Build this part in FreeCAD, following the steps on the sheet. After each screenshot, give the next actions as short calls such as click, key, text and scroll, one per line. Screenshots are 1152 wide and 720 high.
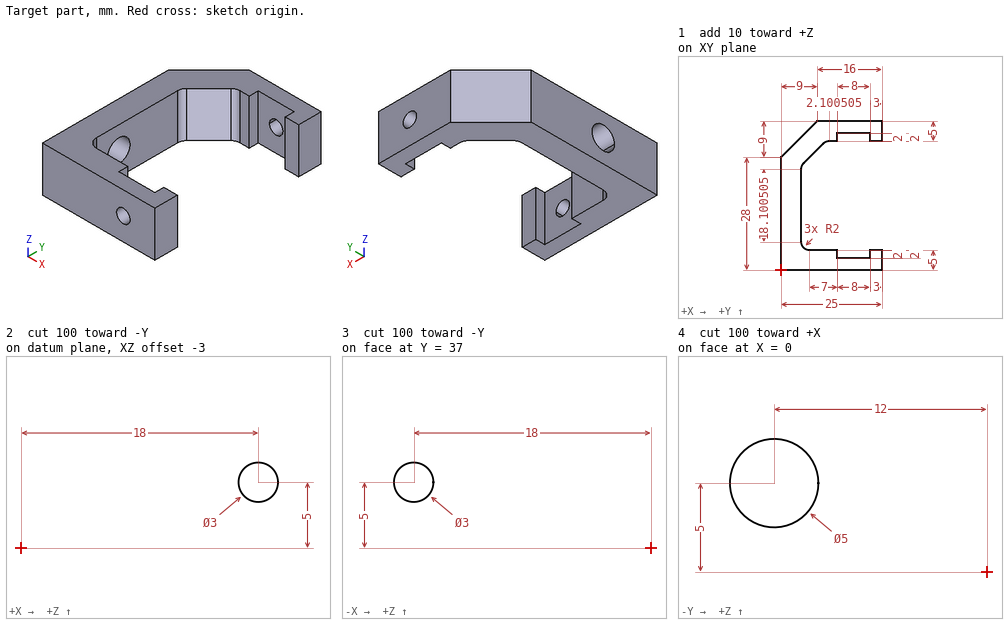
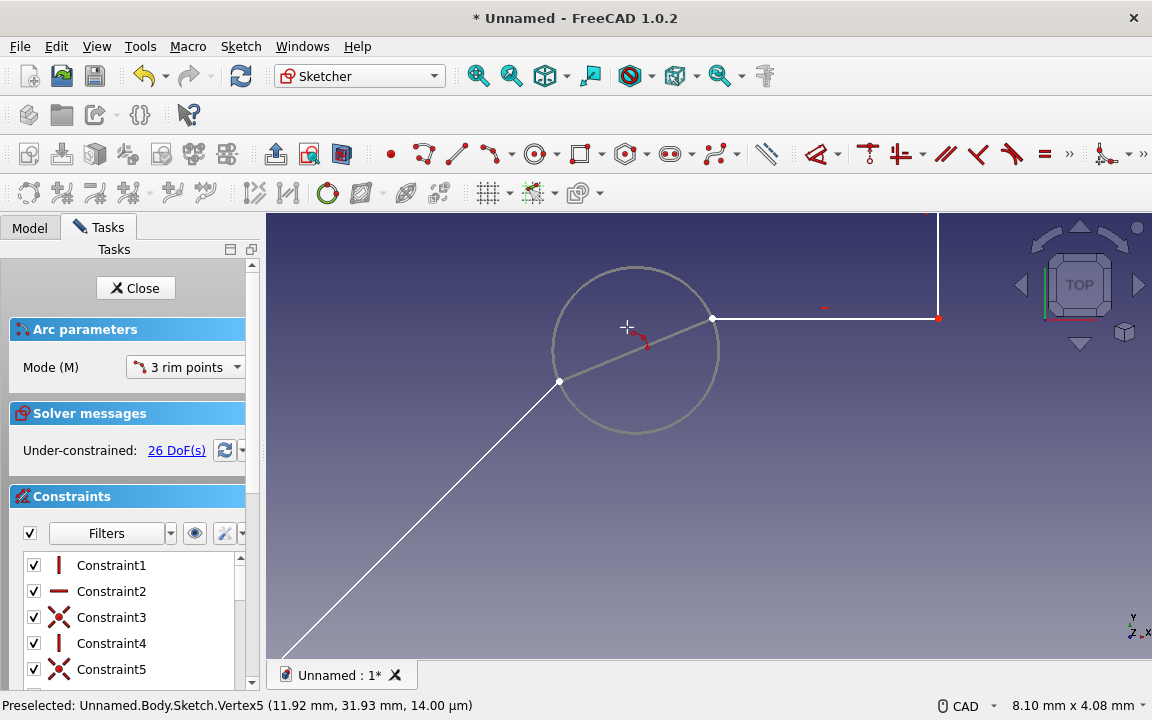
click(627, 328)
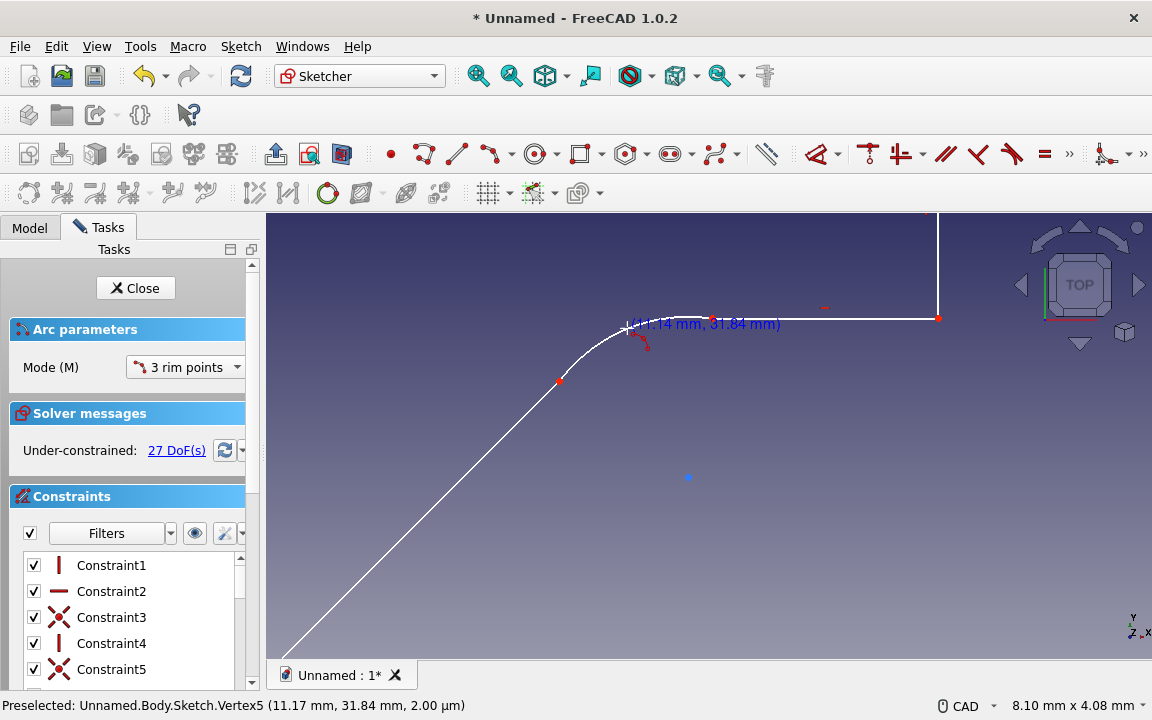
scroll(630, 327, down, 13)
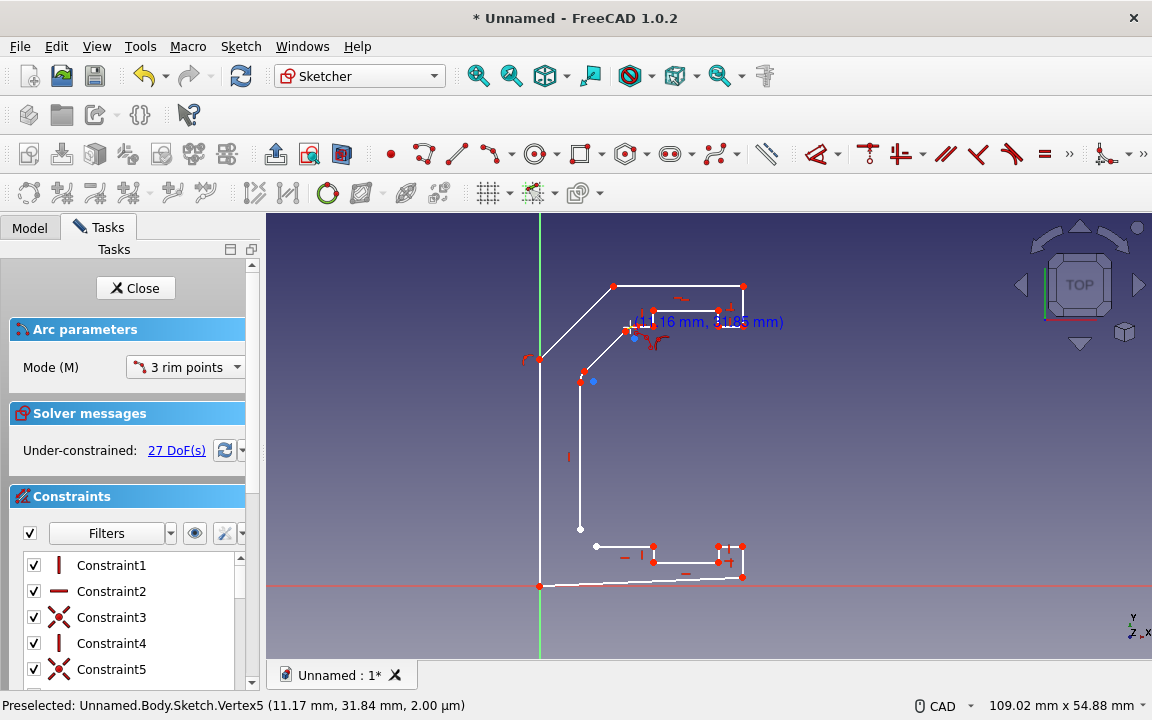
click(597, 547)
click(580, 530)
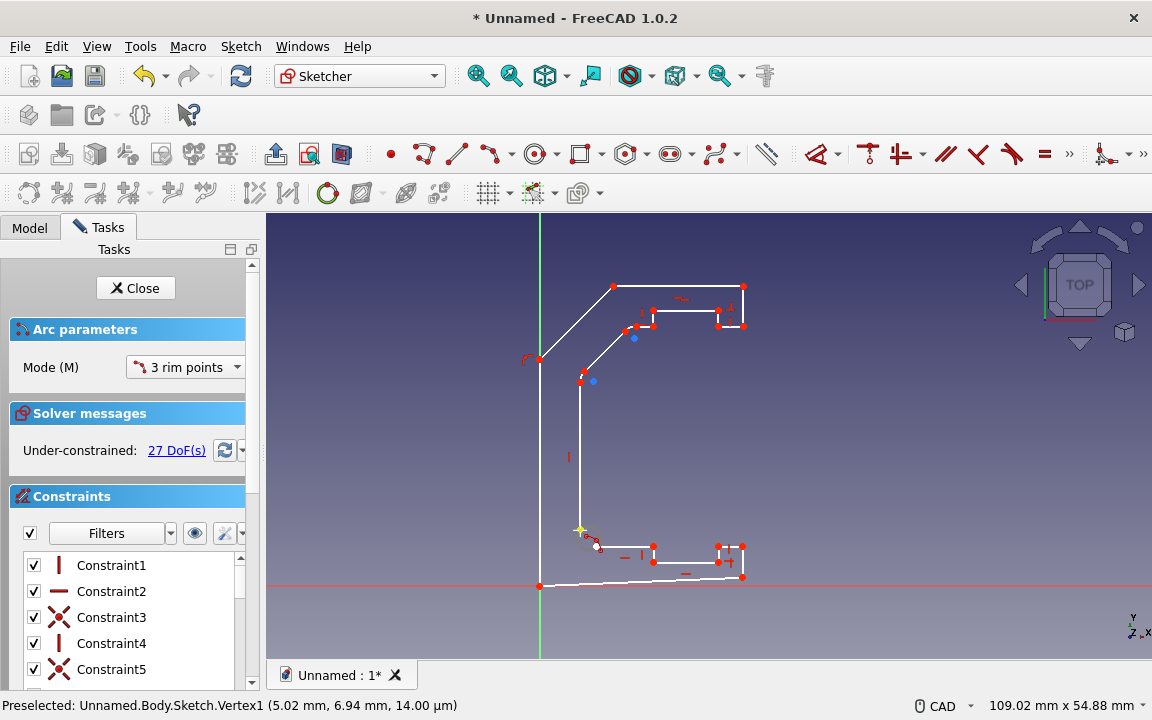
scroll(585, 541, up, 7)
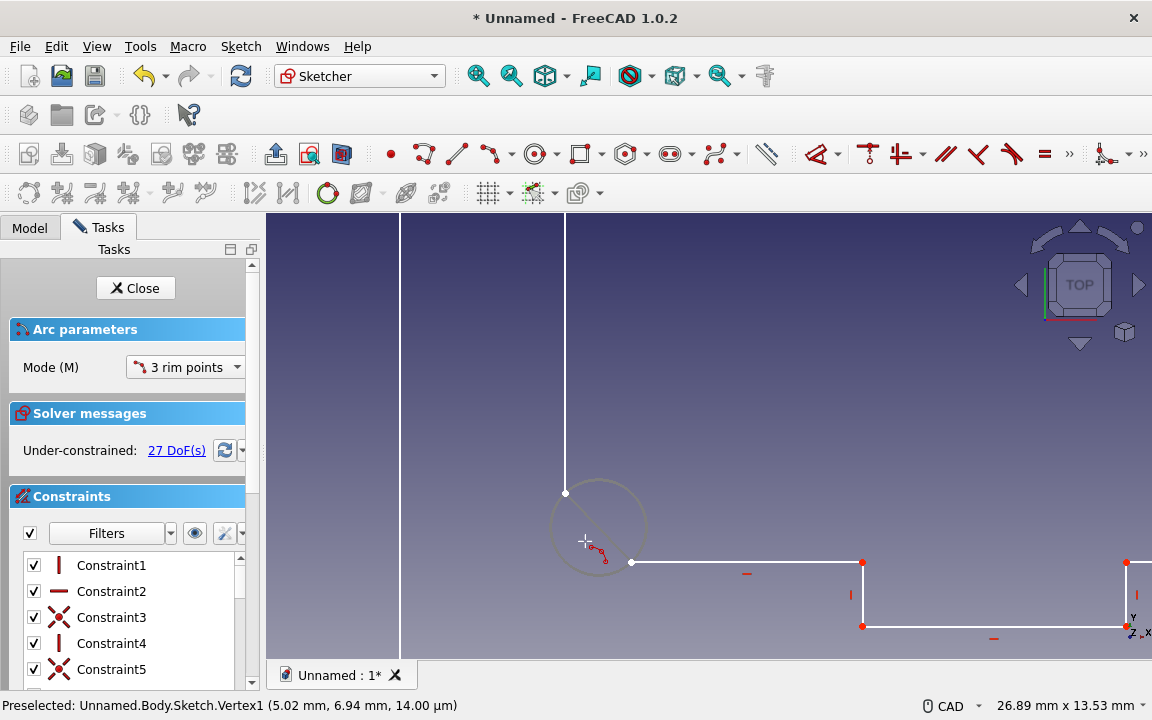
click(584, 538)
key(Escape)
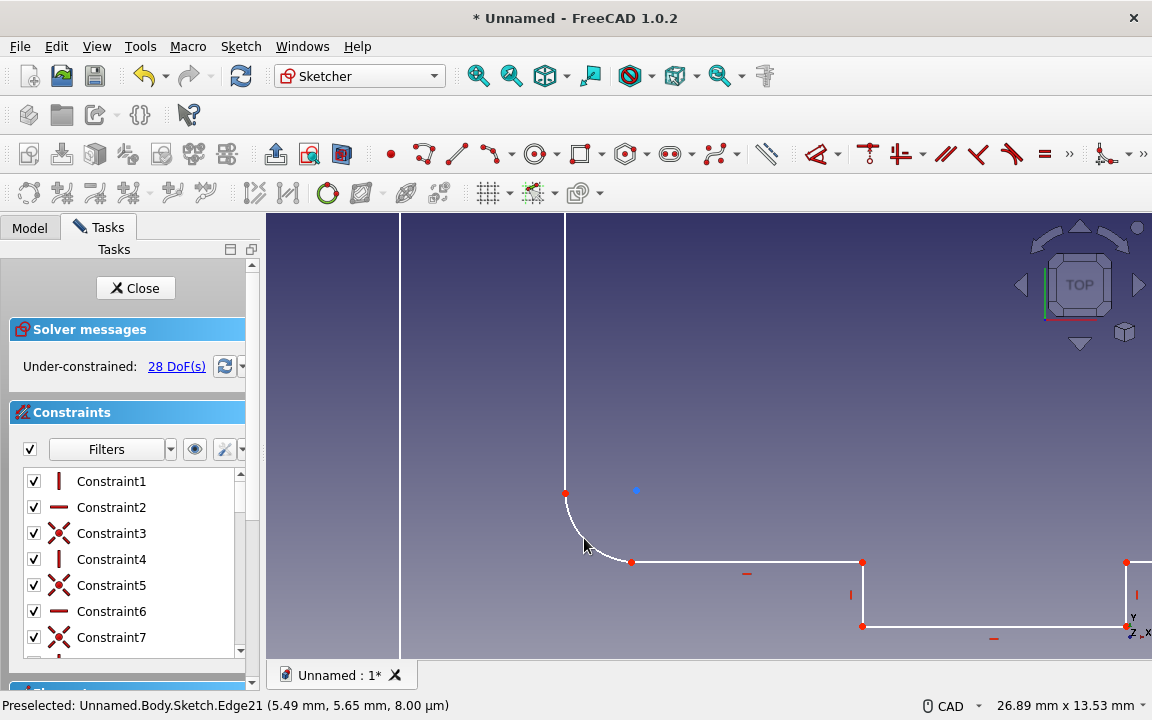
scroll(584, 542, down, 7)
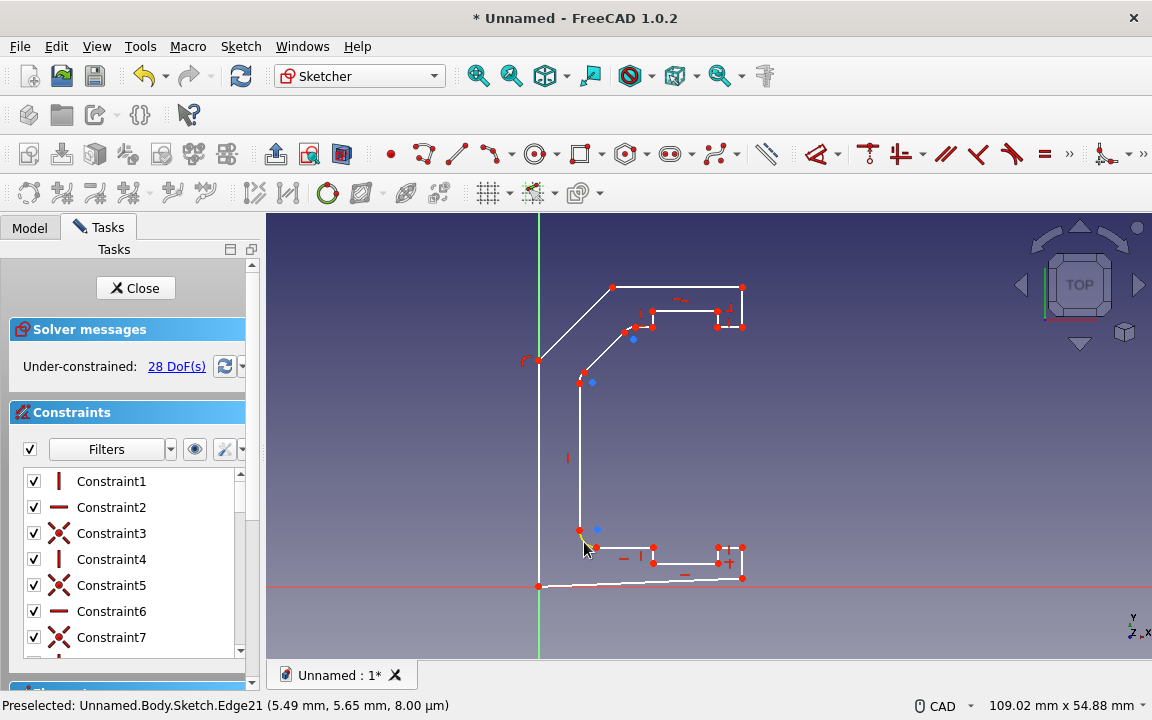
click(580, 486)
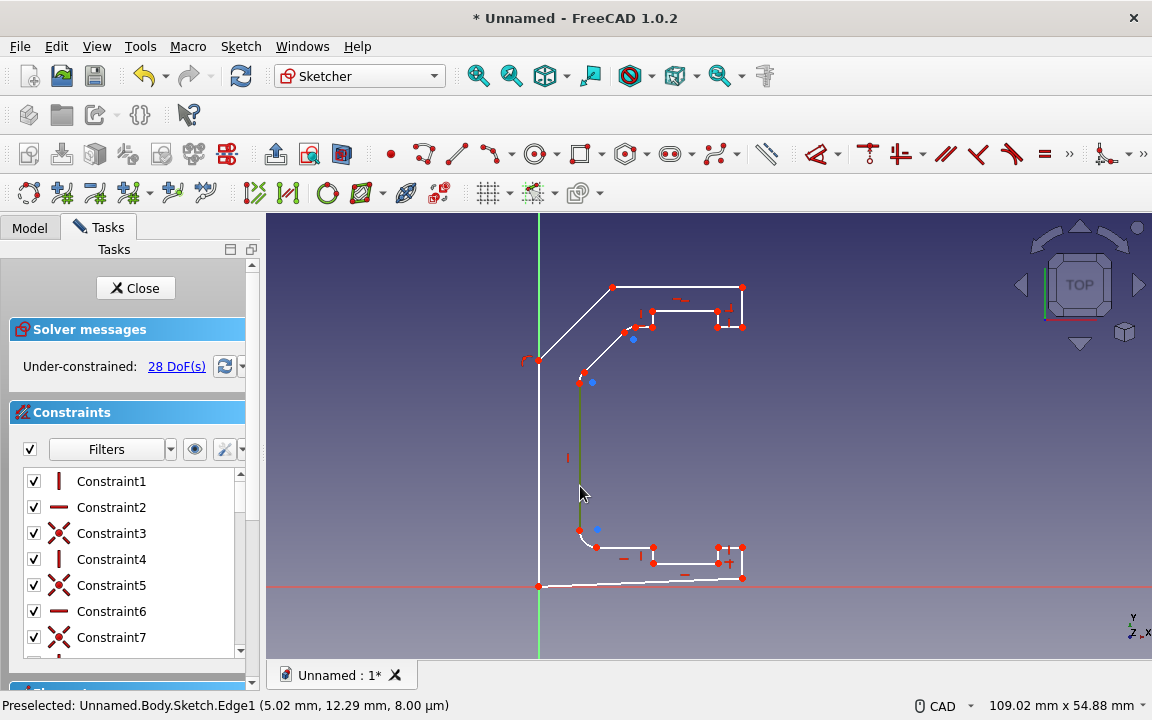
scroll(581, 377, up, 4)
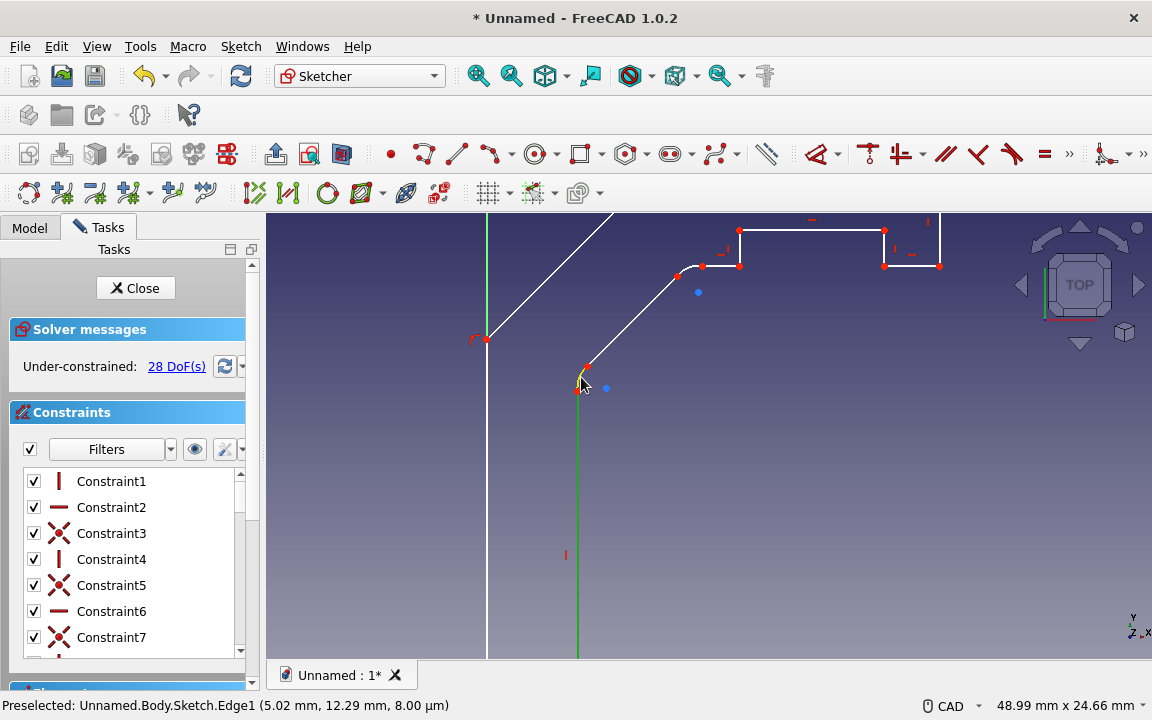
click(580, 377)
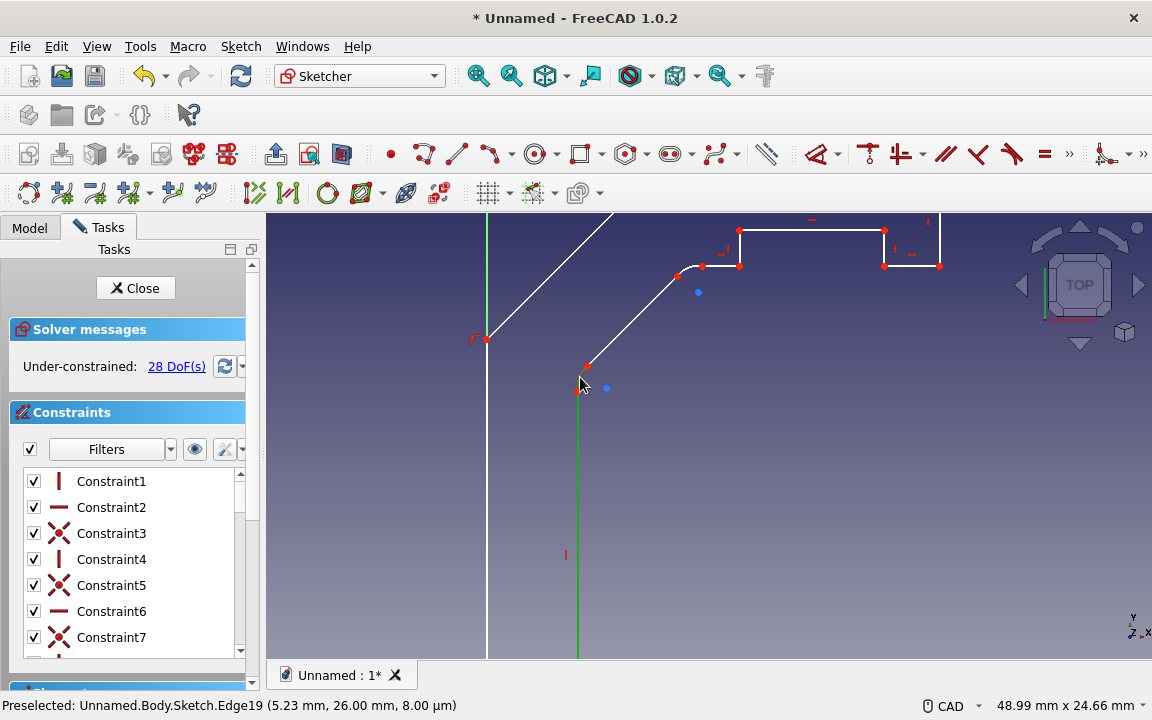
key(t)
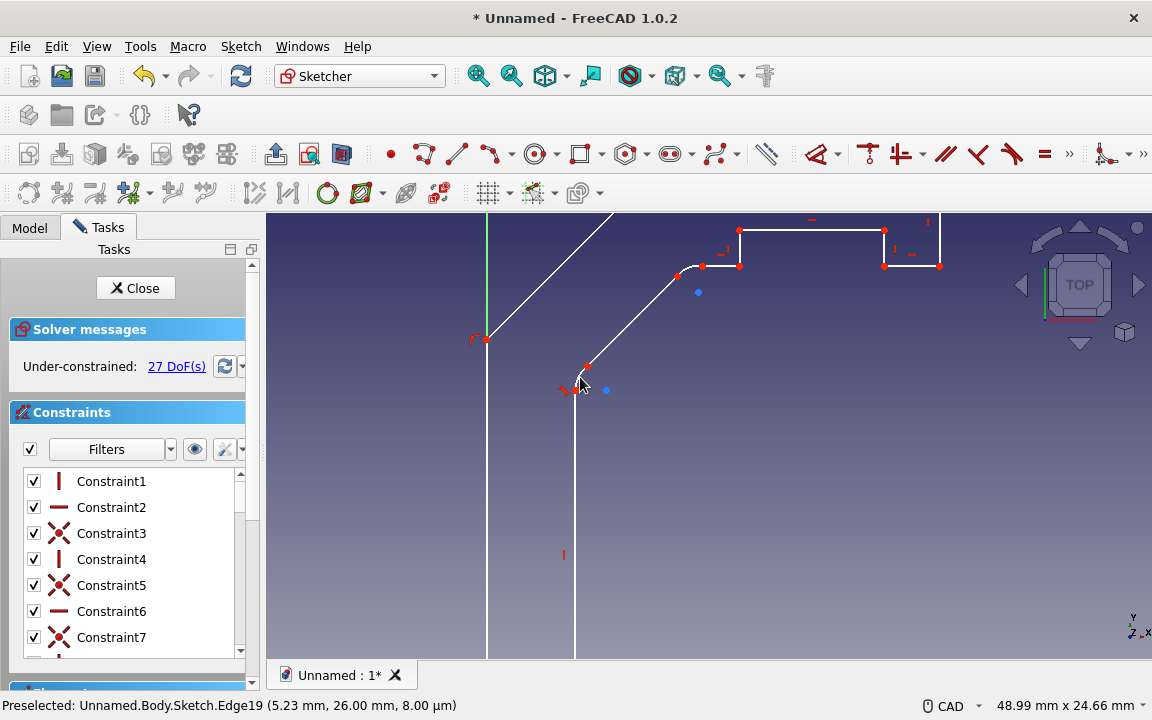
click(575, 620)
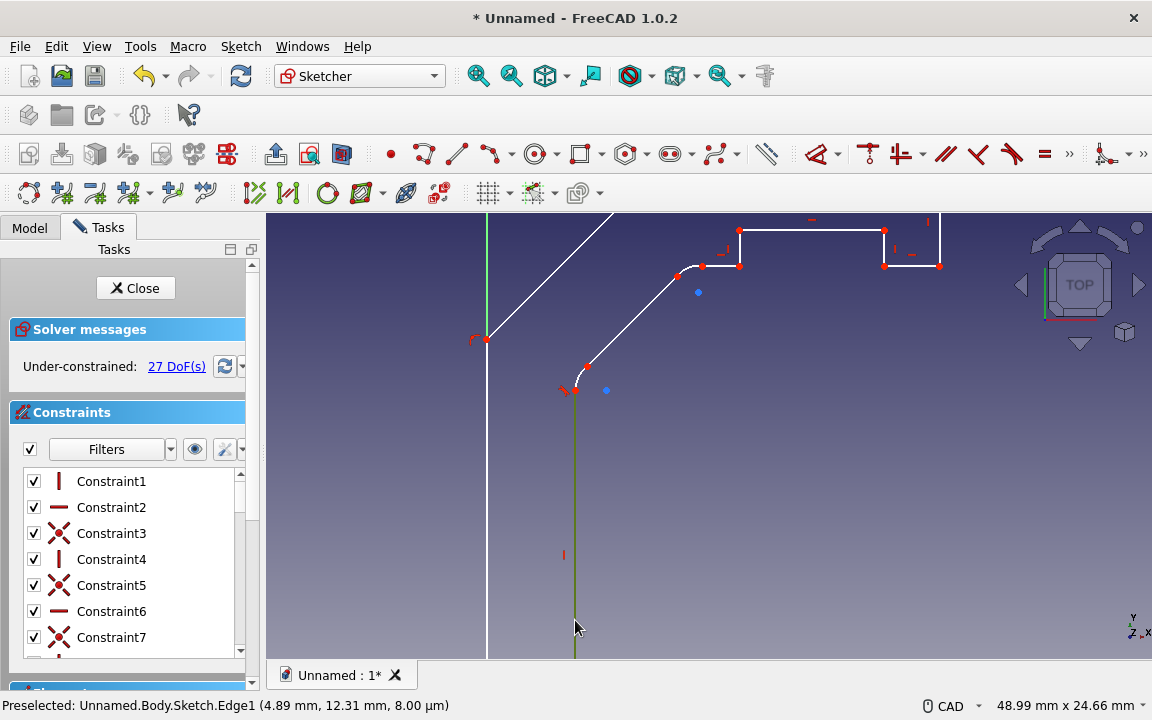
scroll(581, 376, down, 4)